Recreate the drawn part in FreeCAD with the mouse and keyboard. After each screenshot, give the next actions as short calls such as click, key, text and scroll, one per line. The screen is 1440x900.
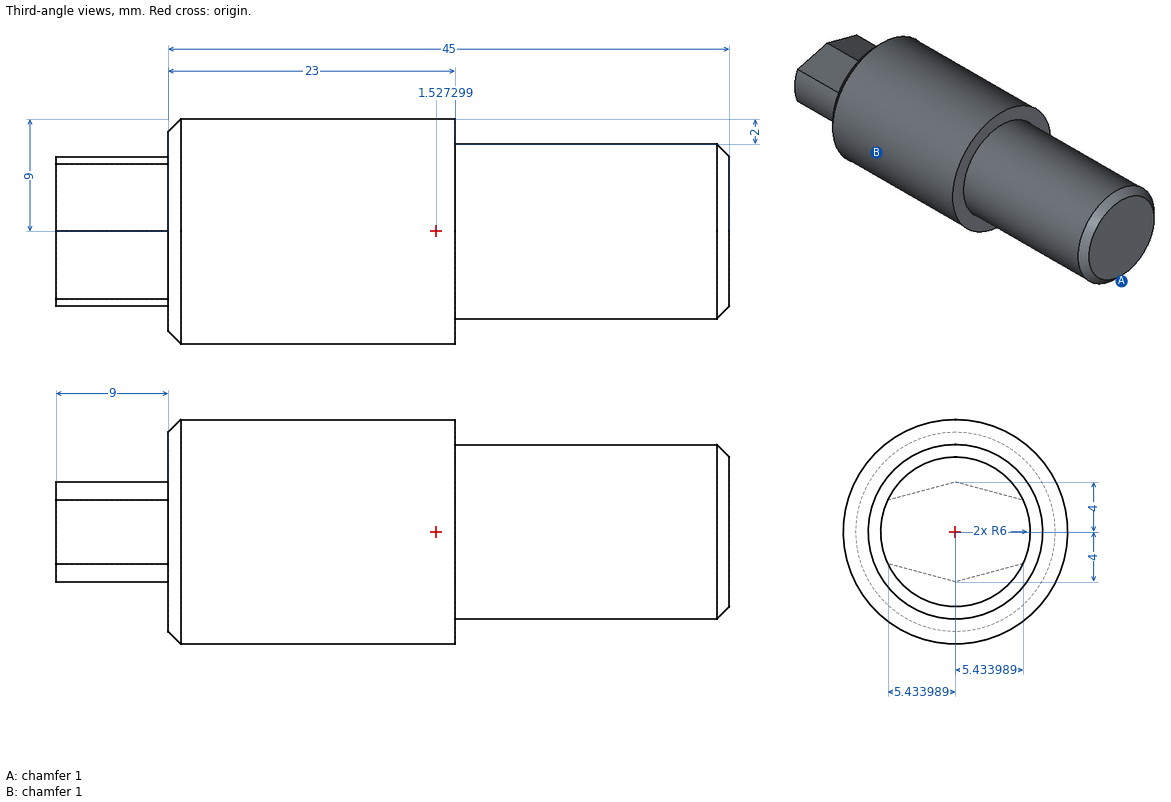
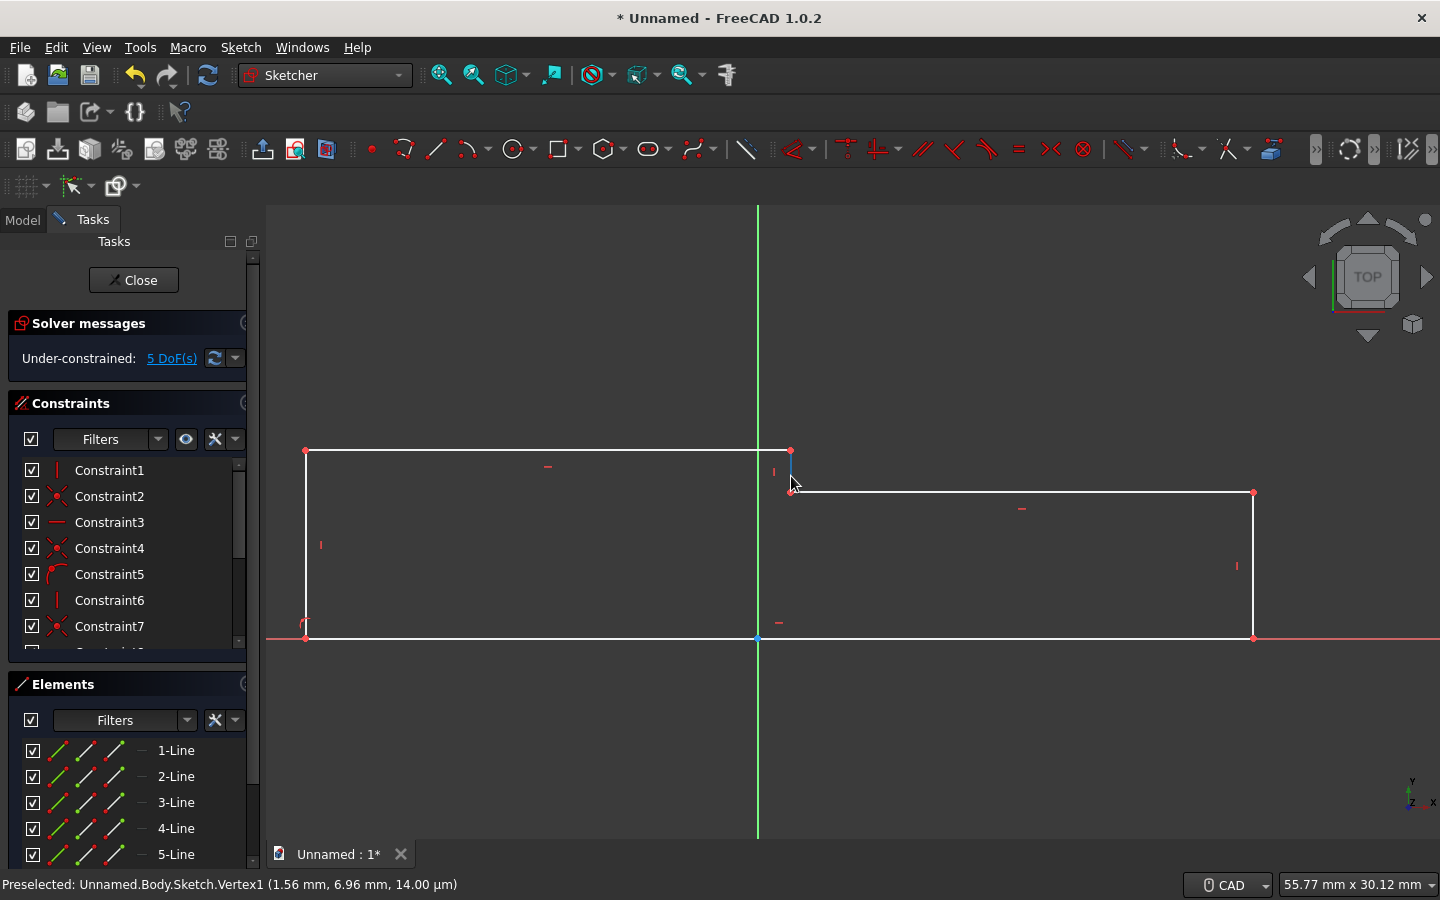
click(791, 475)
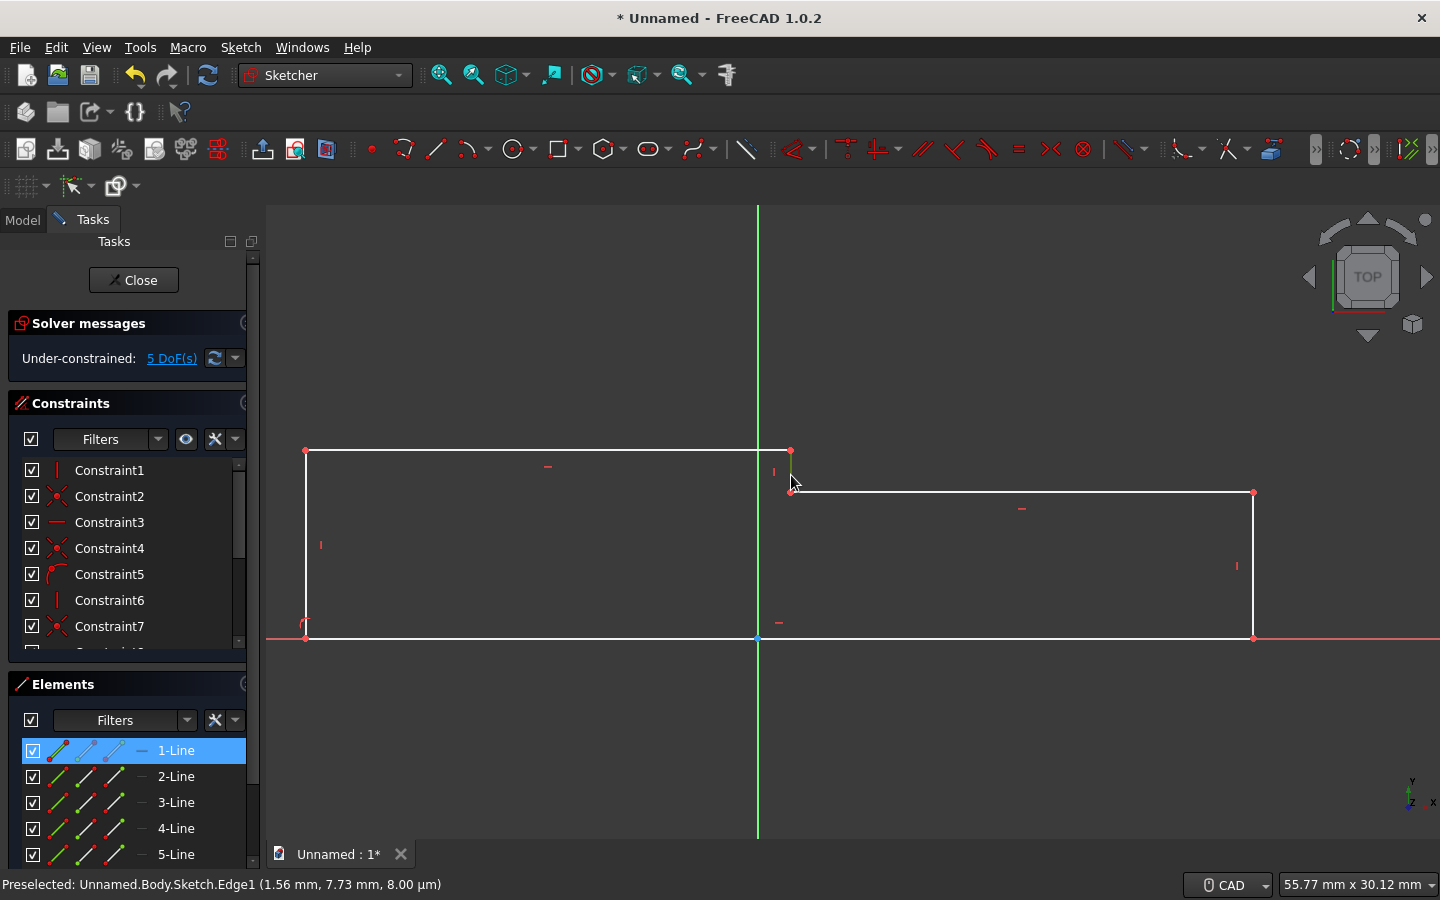
click(814, 150)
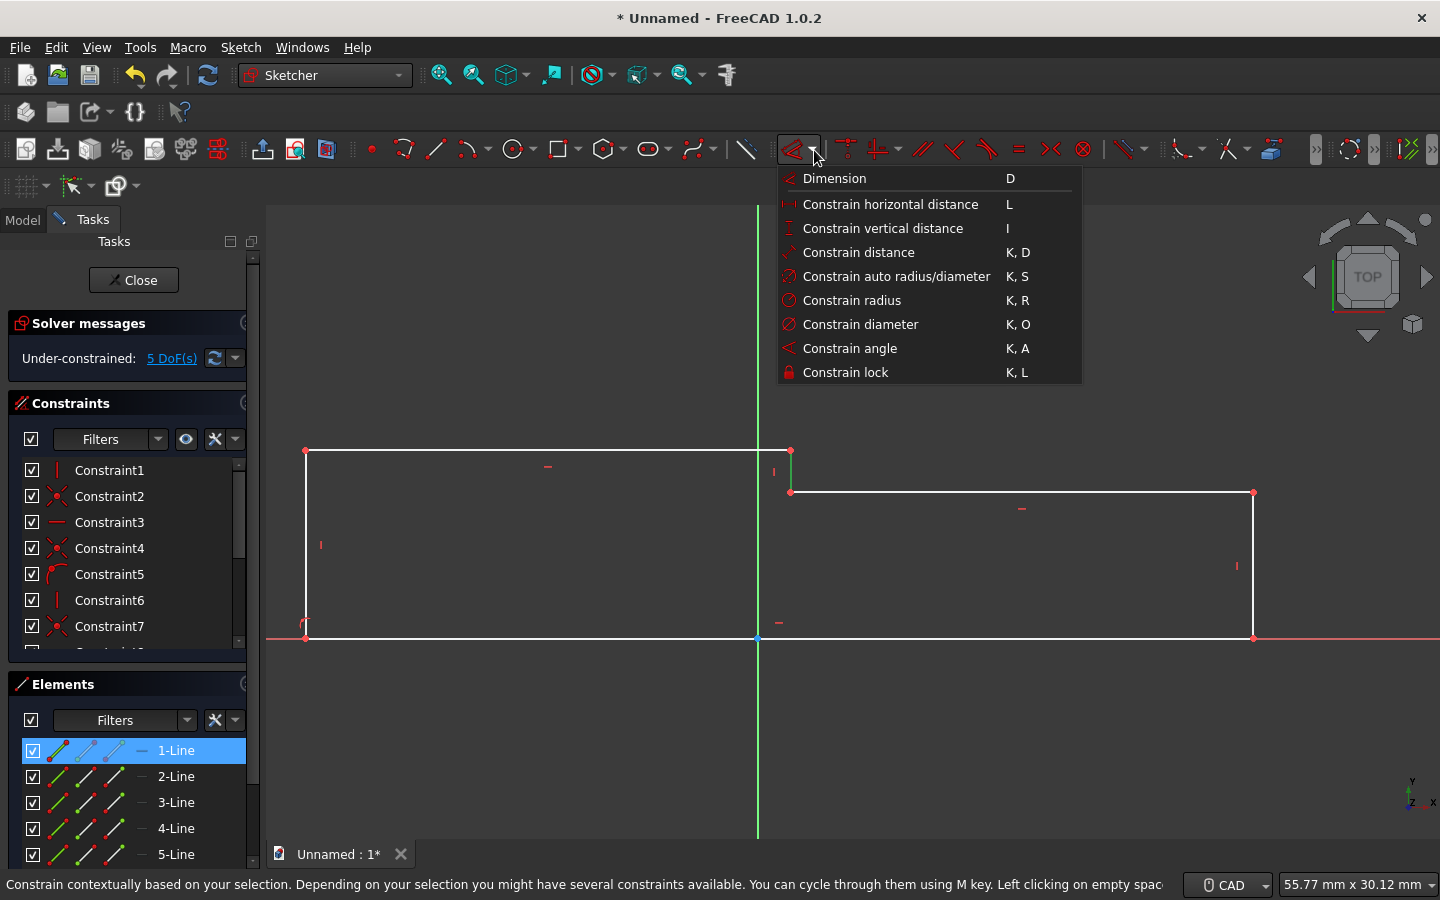
click(930, 228)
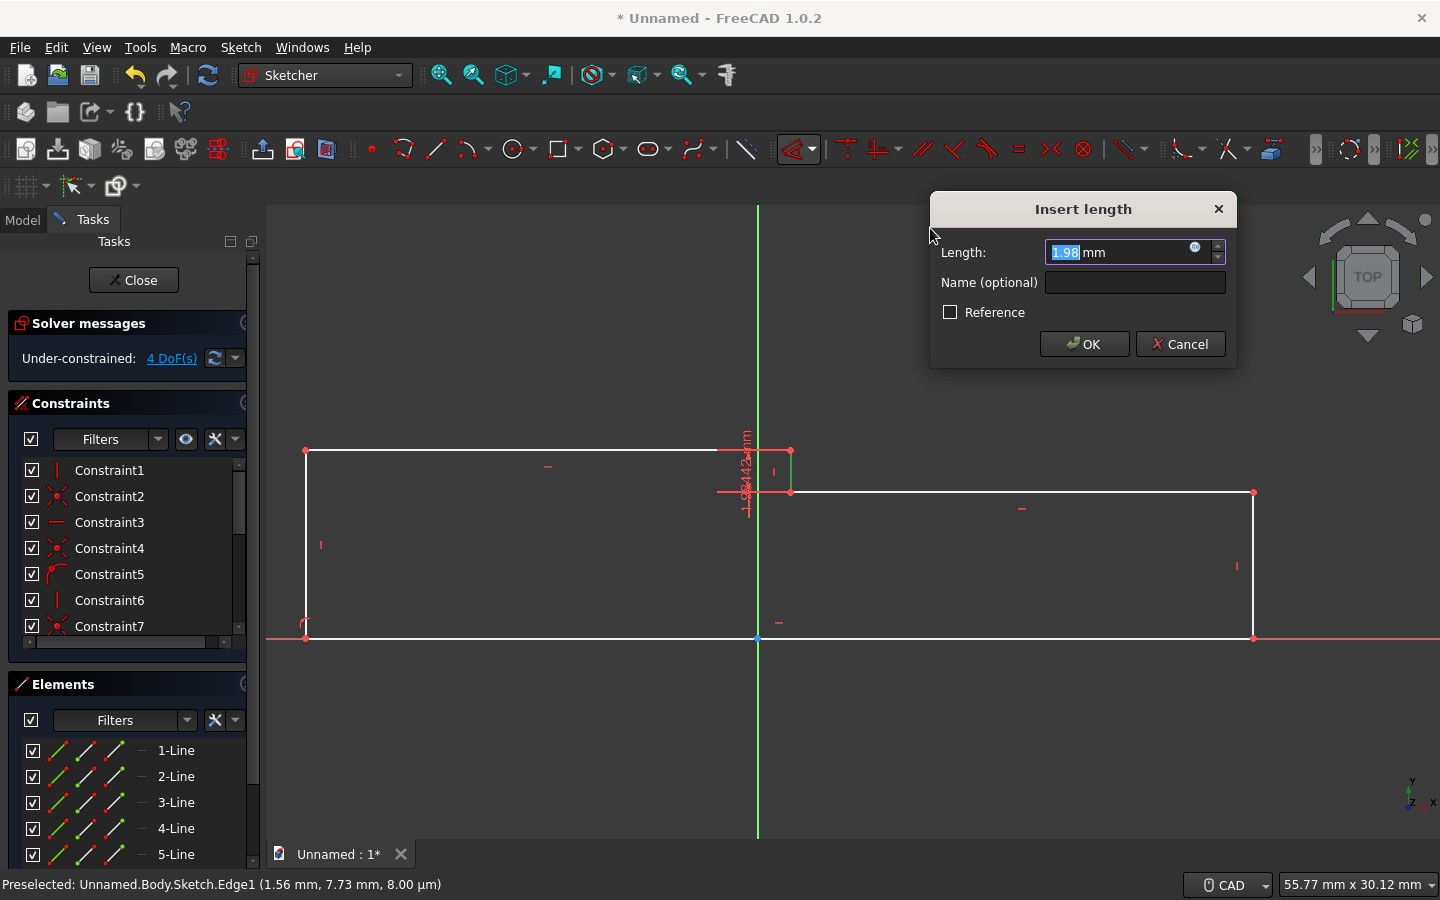
text(2)
key(Return)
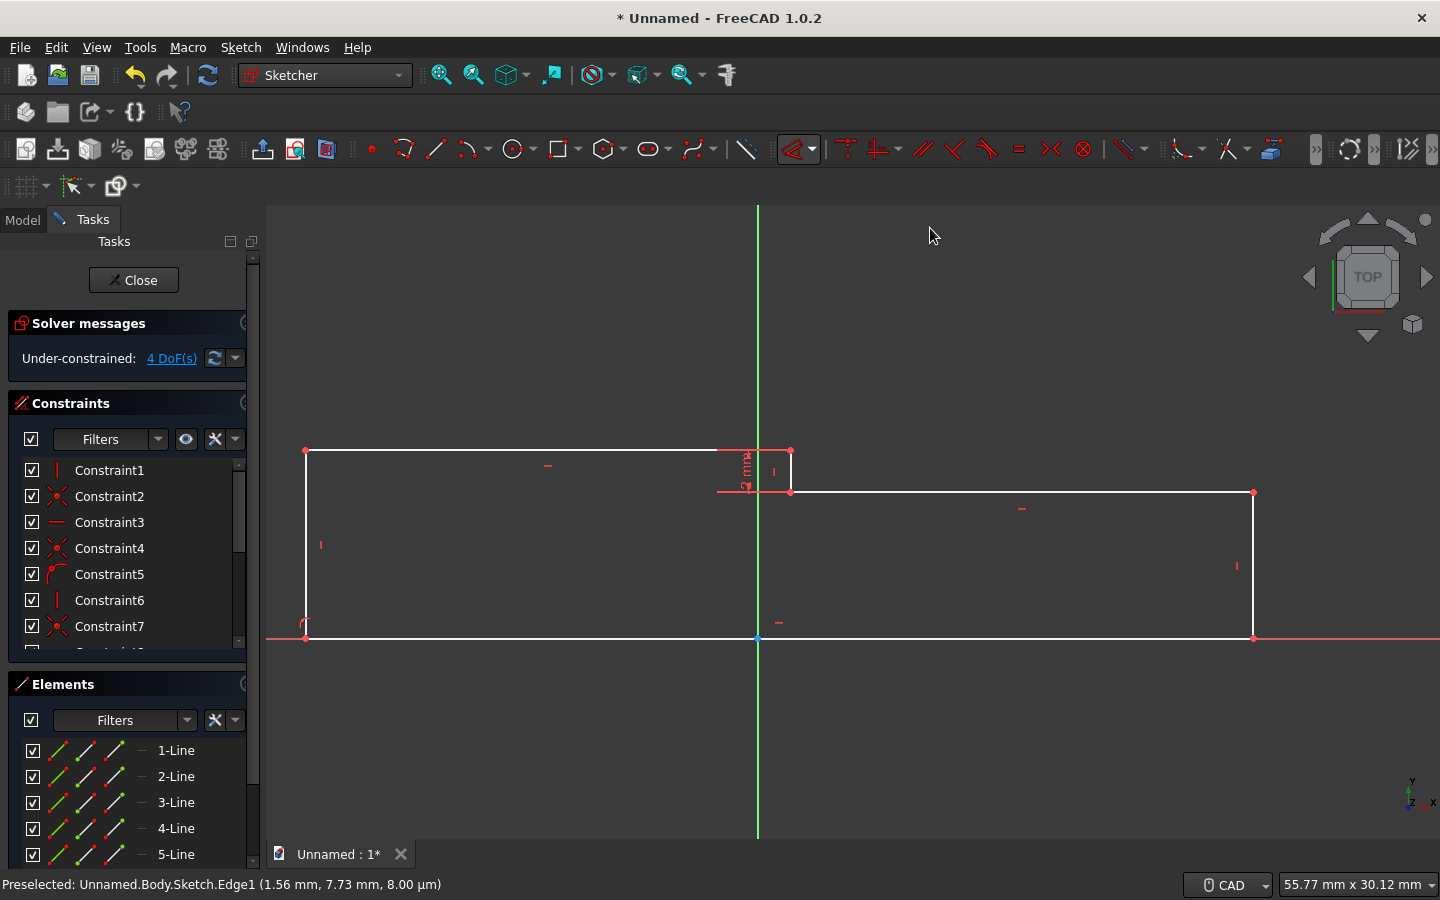
click(306, 507)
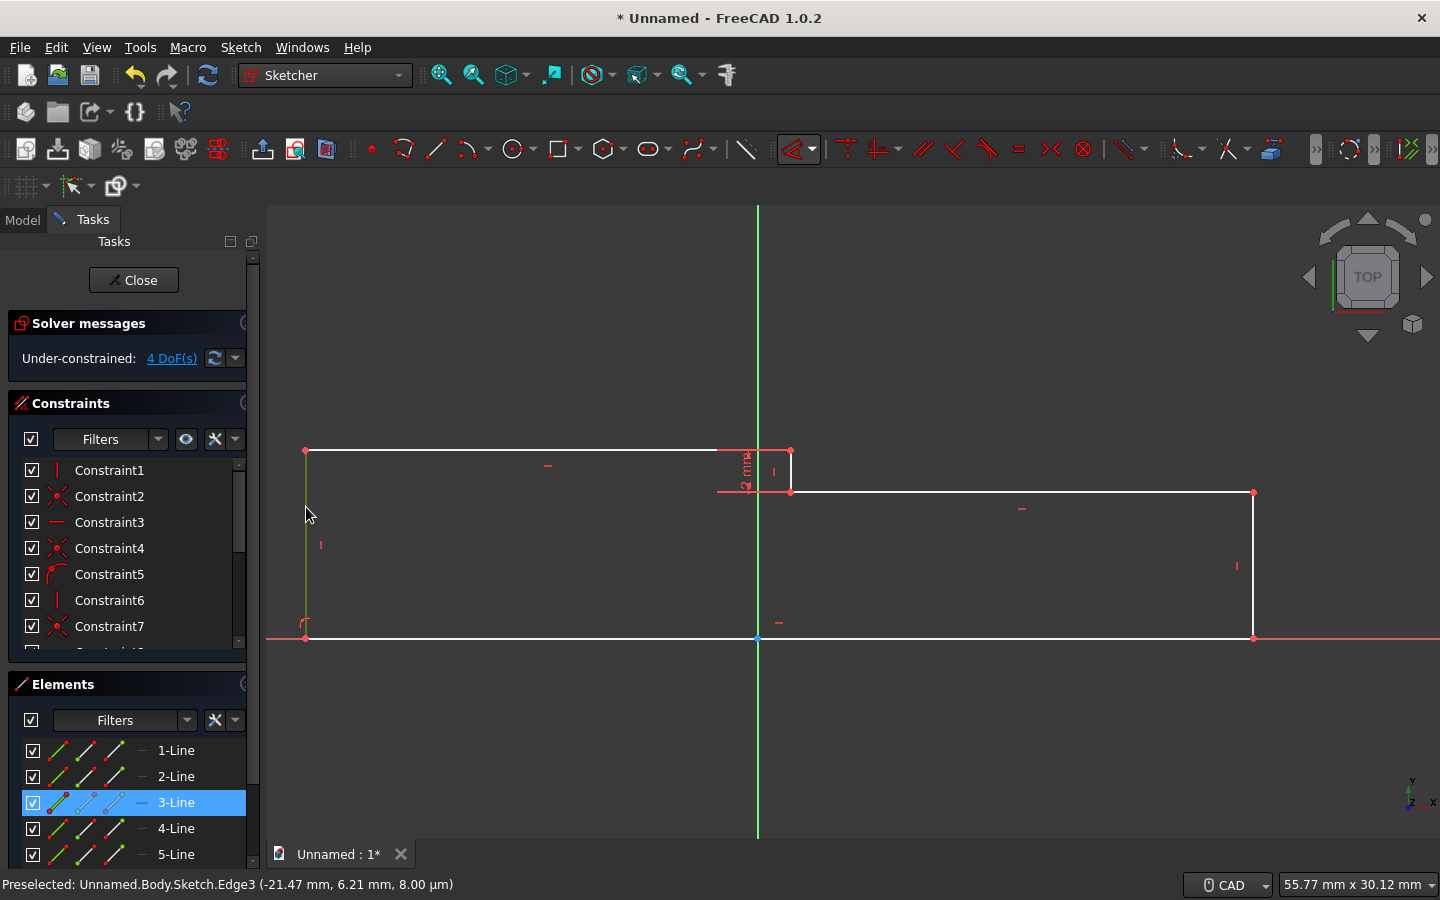
click(814, 150)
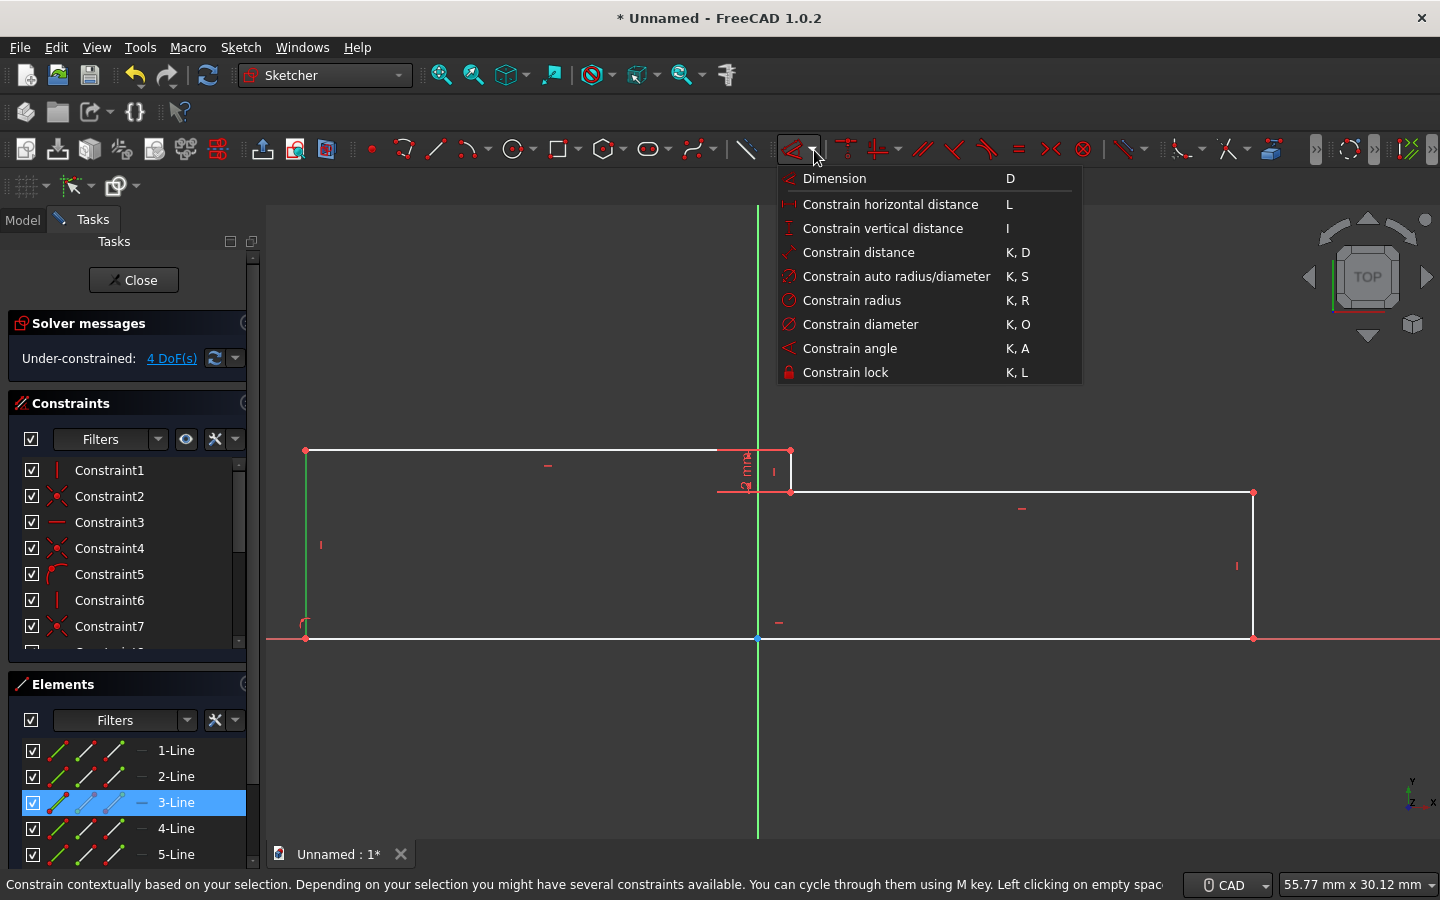
click(930, 228)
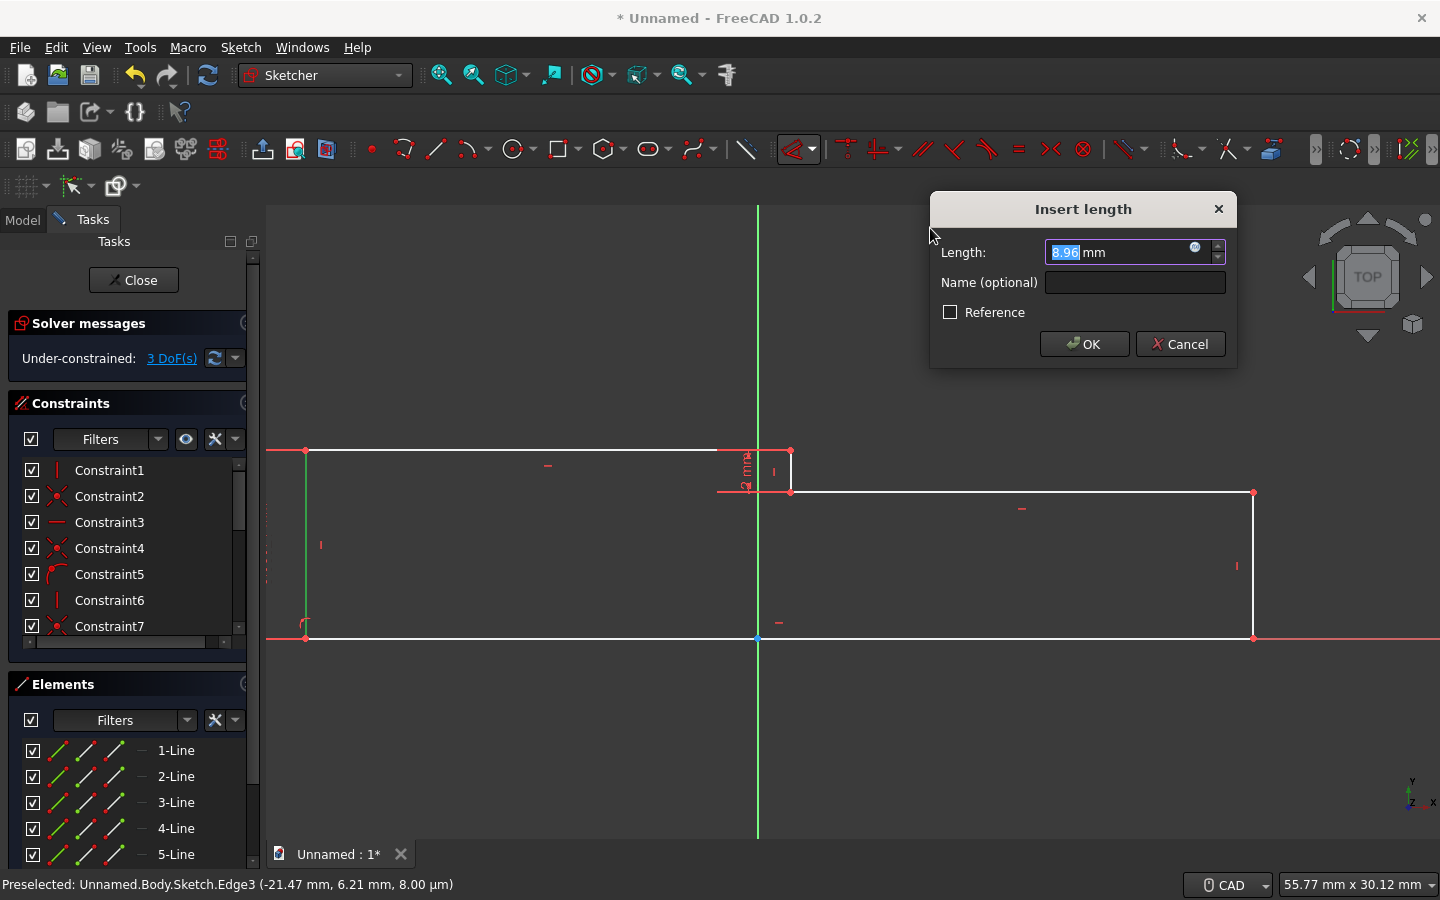
text(9)
key(Return)